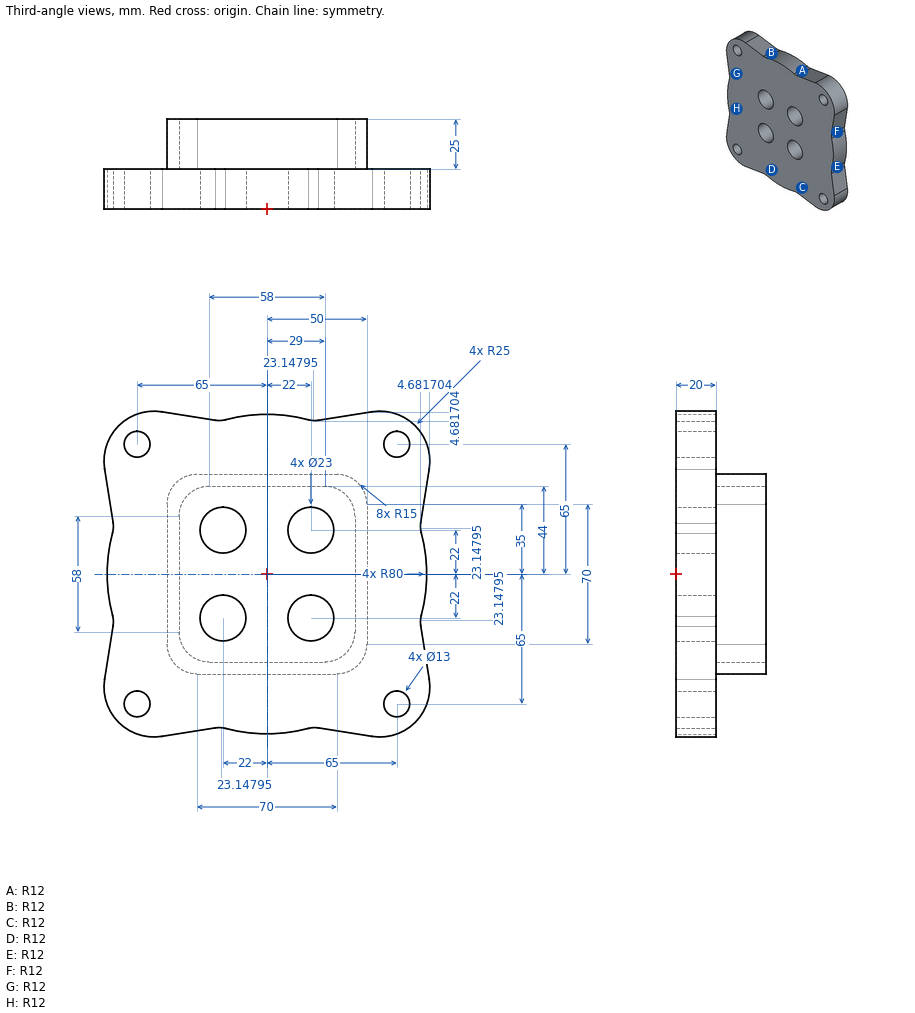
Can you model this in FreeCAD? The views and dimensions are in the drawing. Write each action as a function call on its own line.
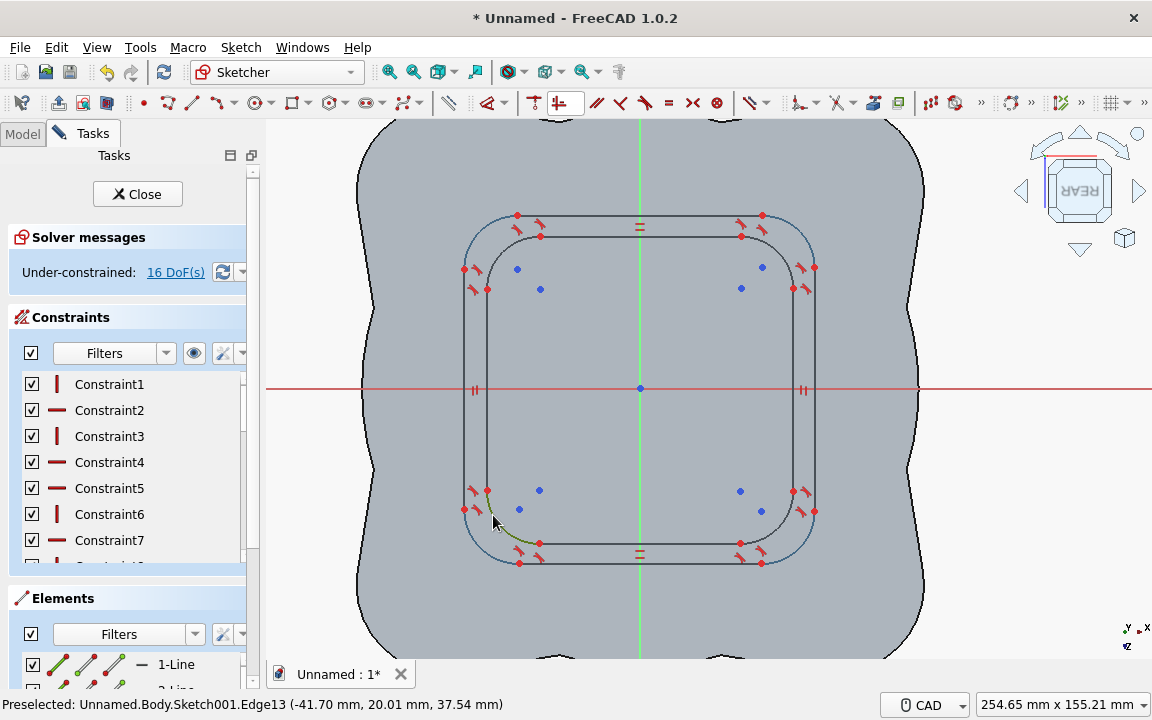
click(516, 243)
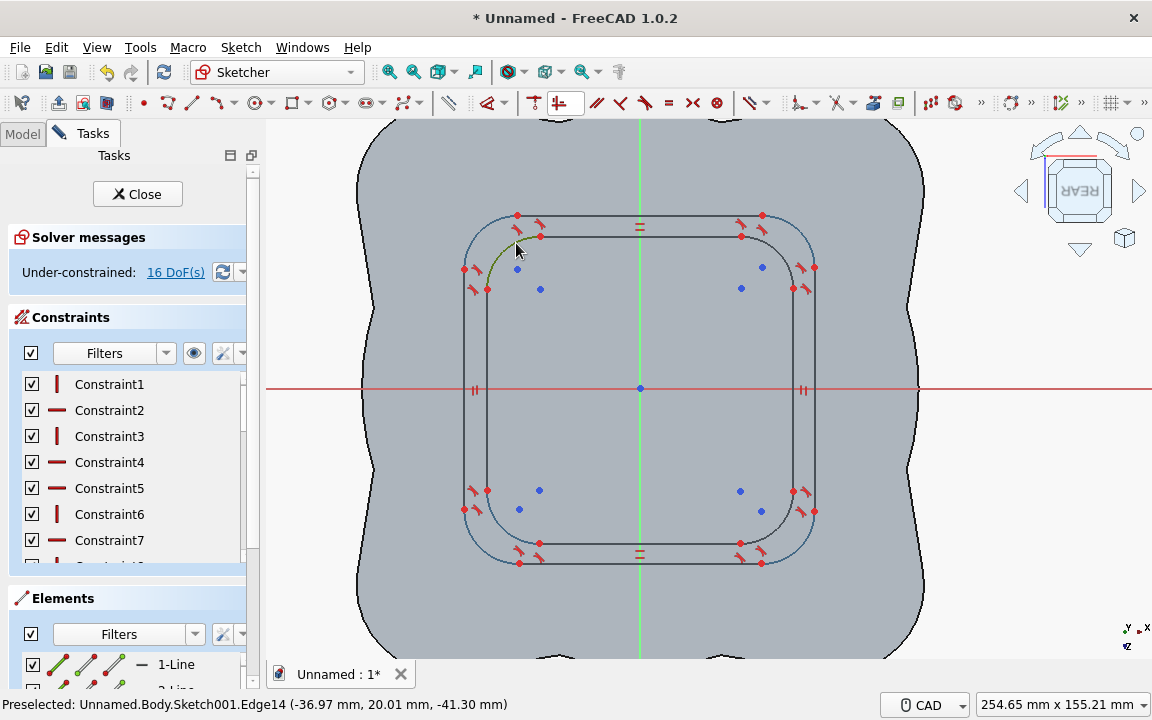
click(788, 265)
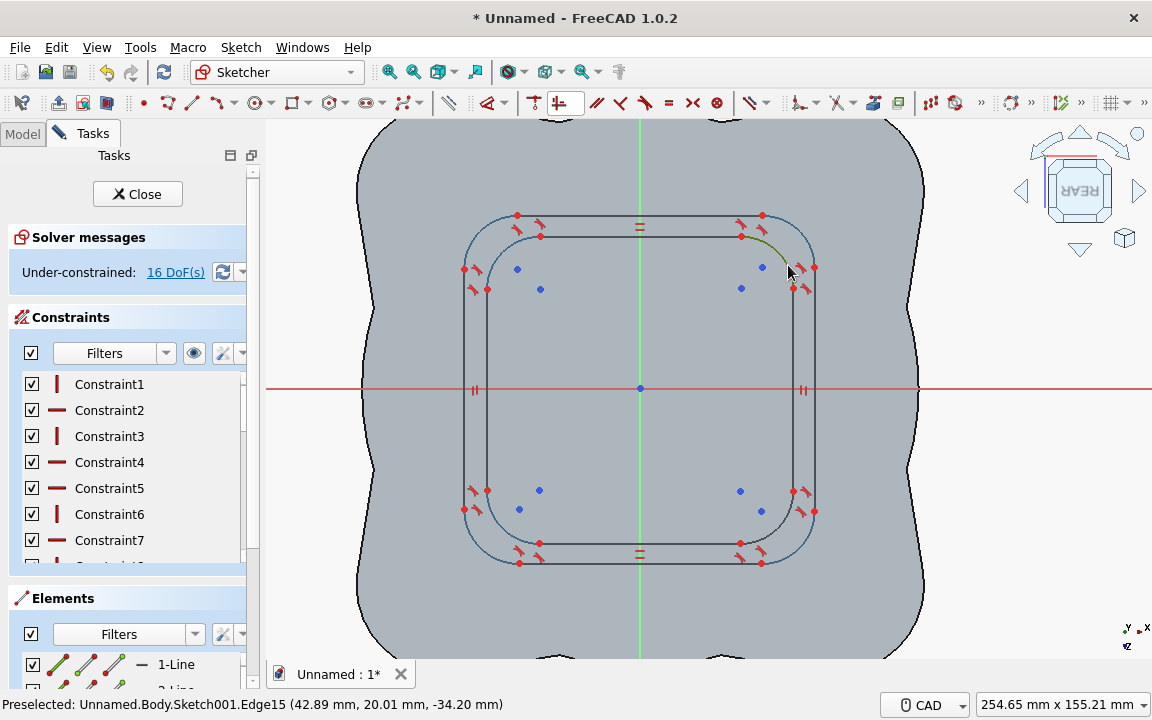
click(764, 538)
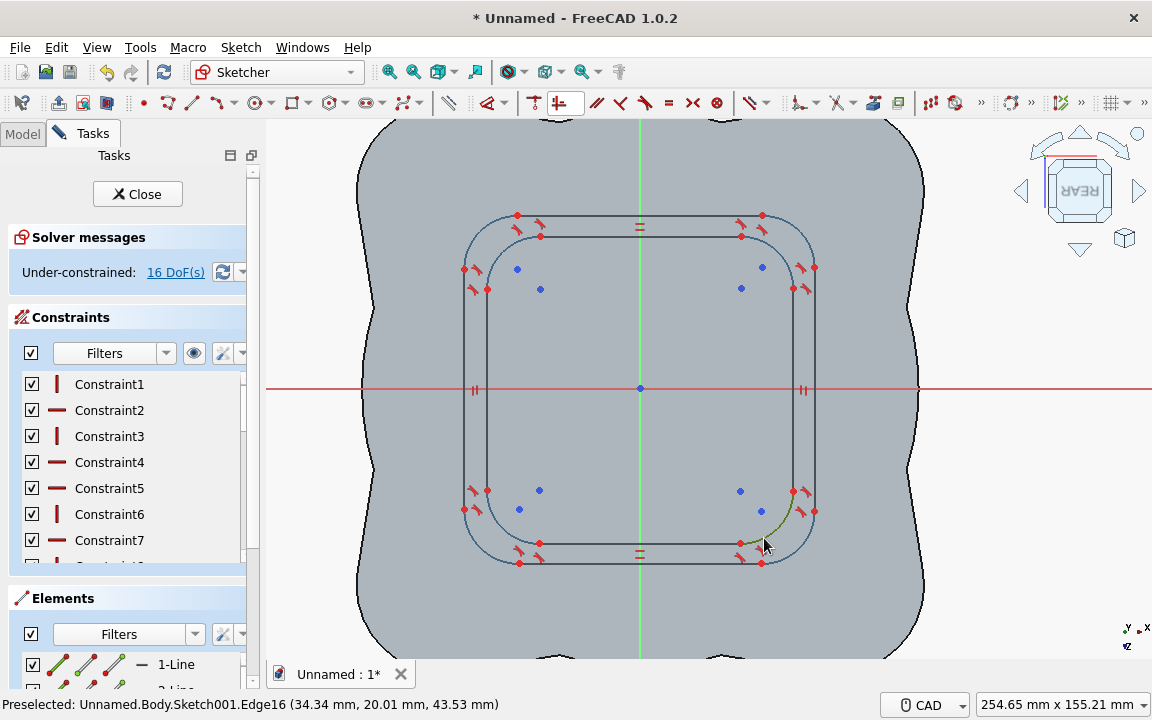
click(670, 104)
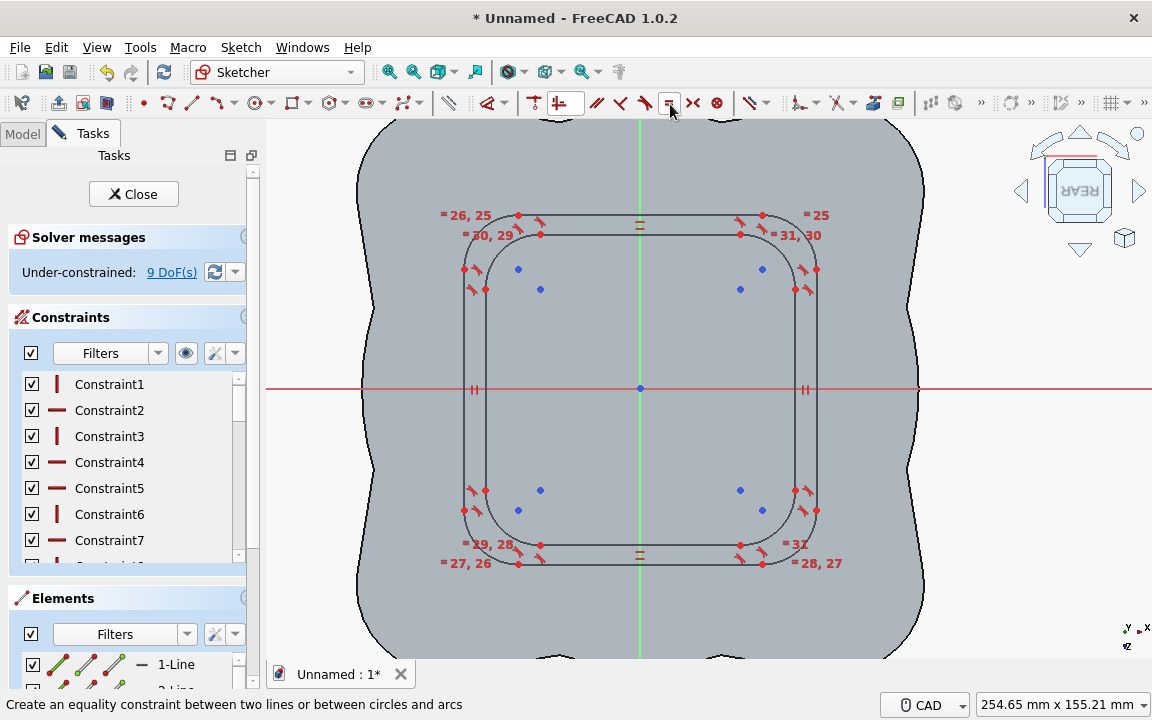
click(488, 104)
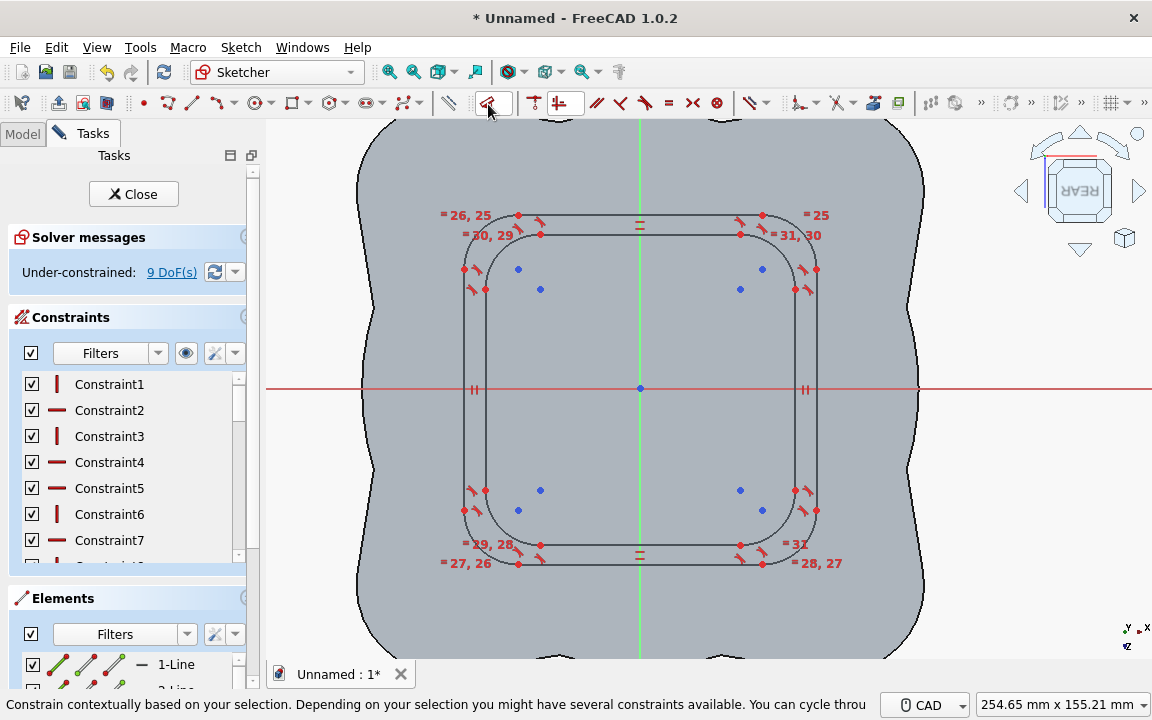
click(811, 245)
click(840, 231)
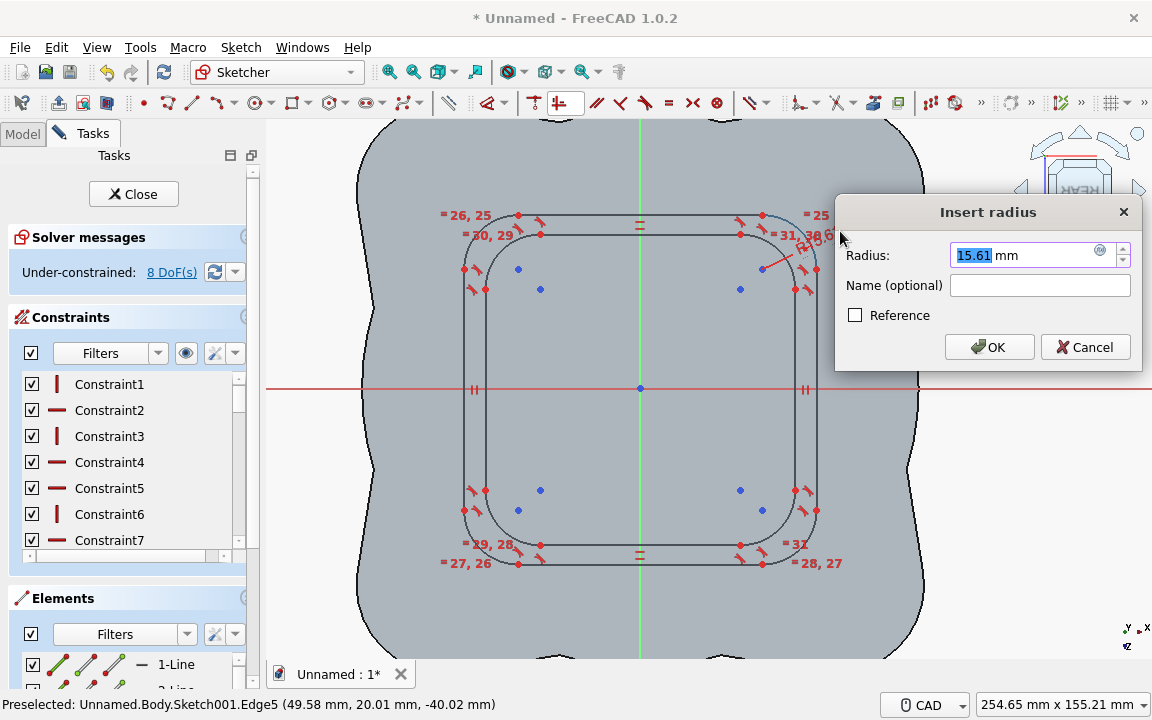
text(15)
key(Return)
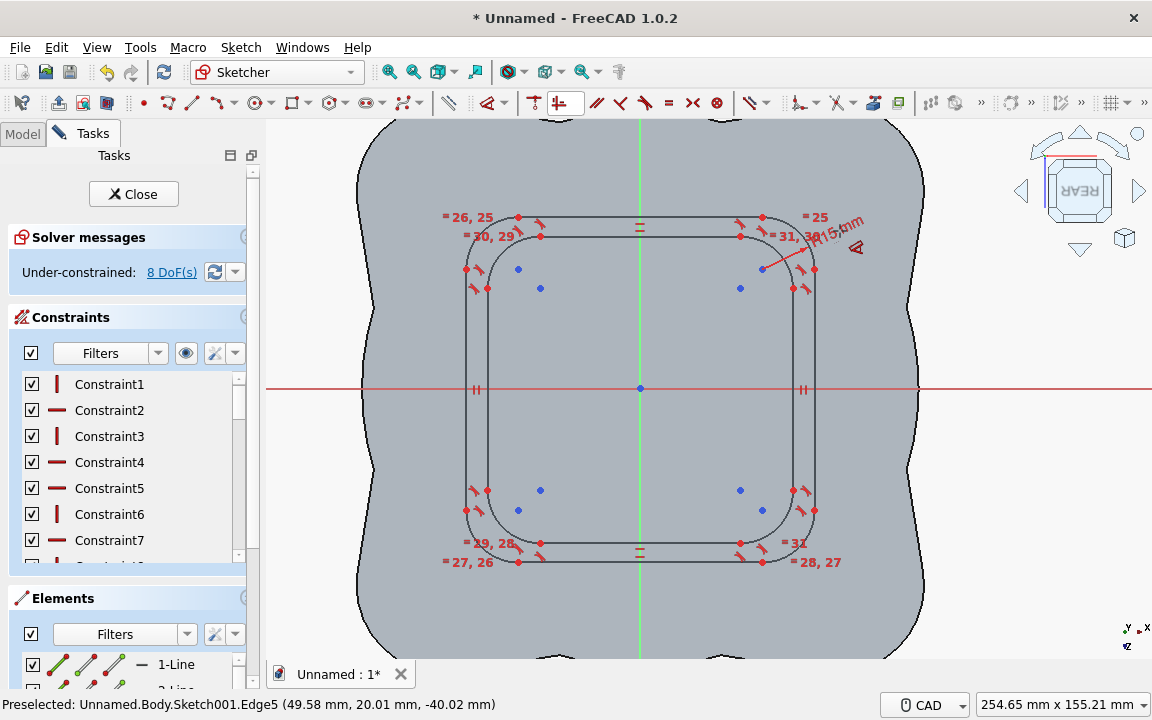
click(815, 438)
click(849, 335)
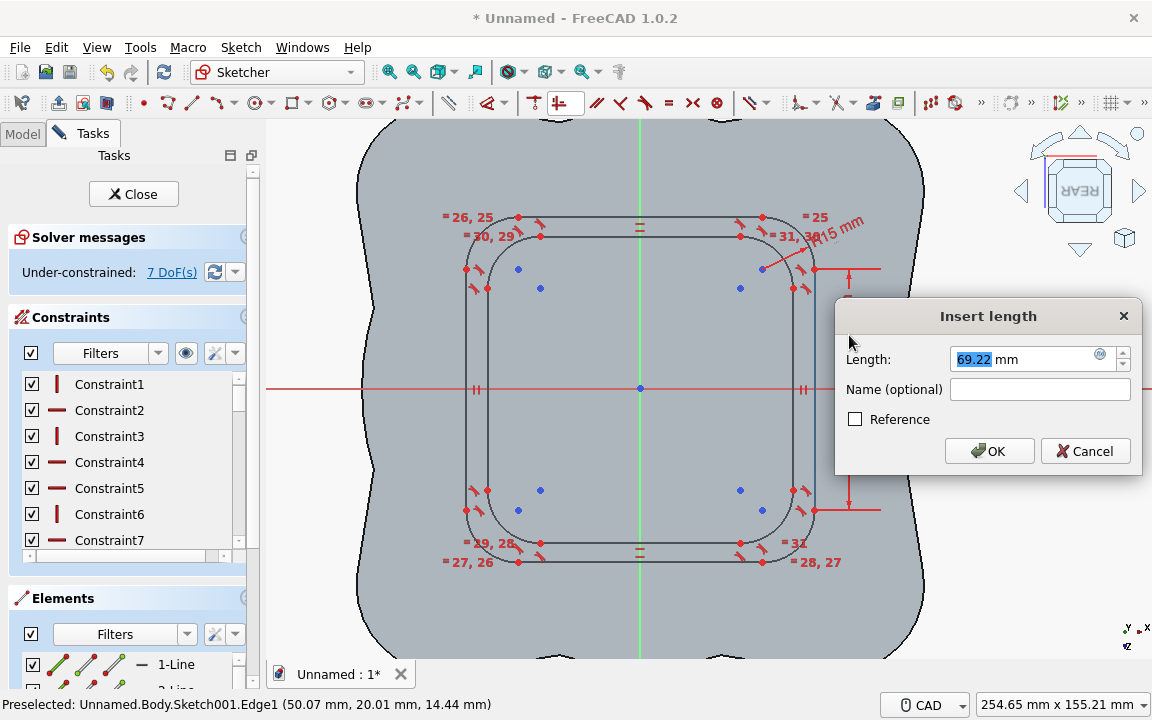
text(70)
key(Return)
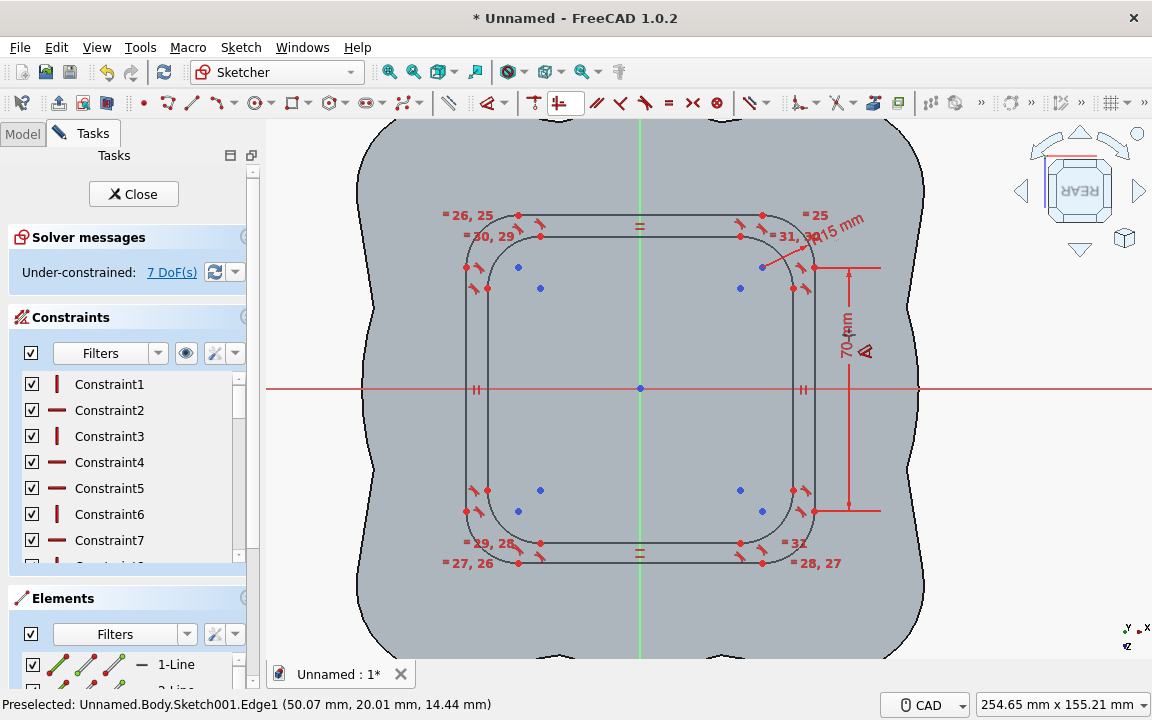
click(689, 215)
click(584, 181)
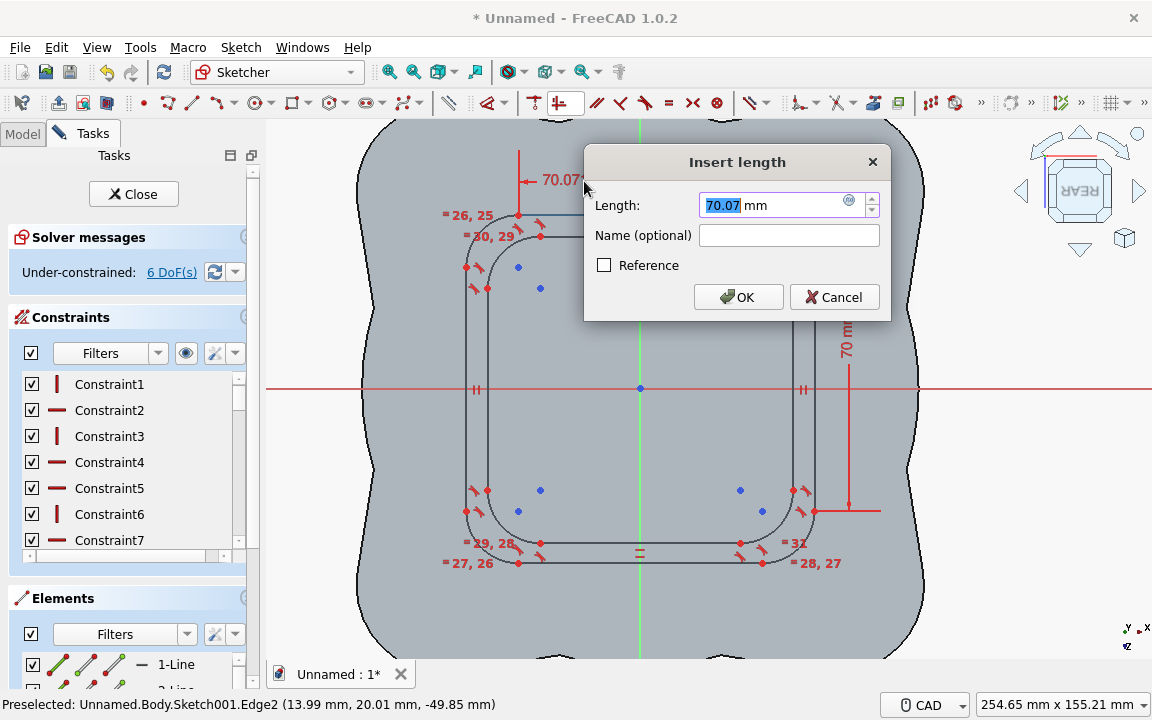
text(70)
key(Return)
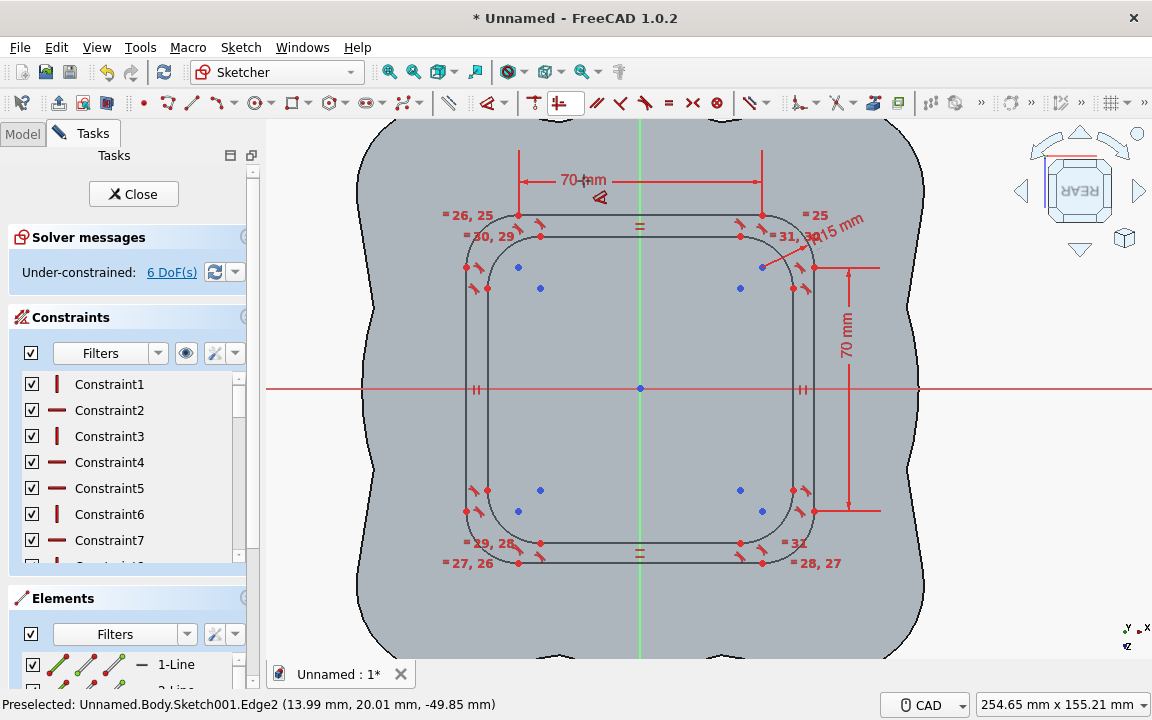
click(681, 543)
click(594, 577)